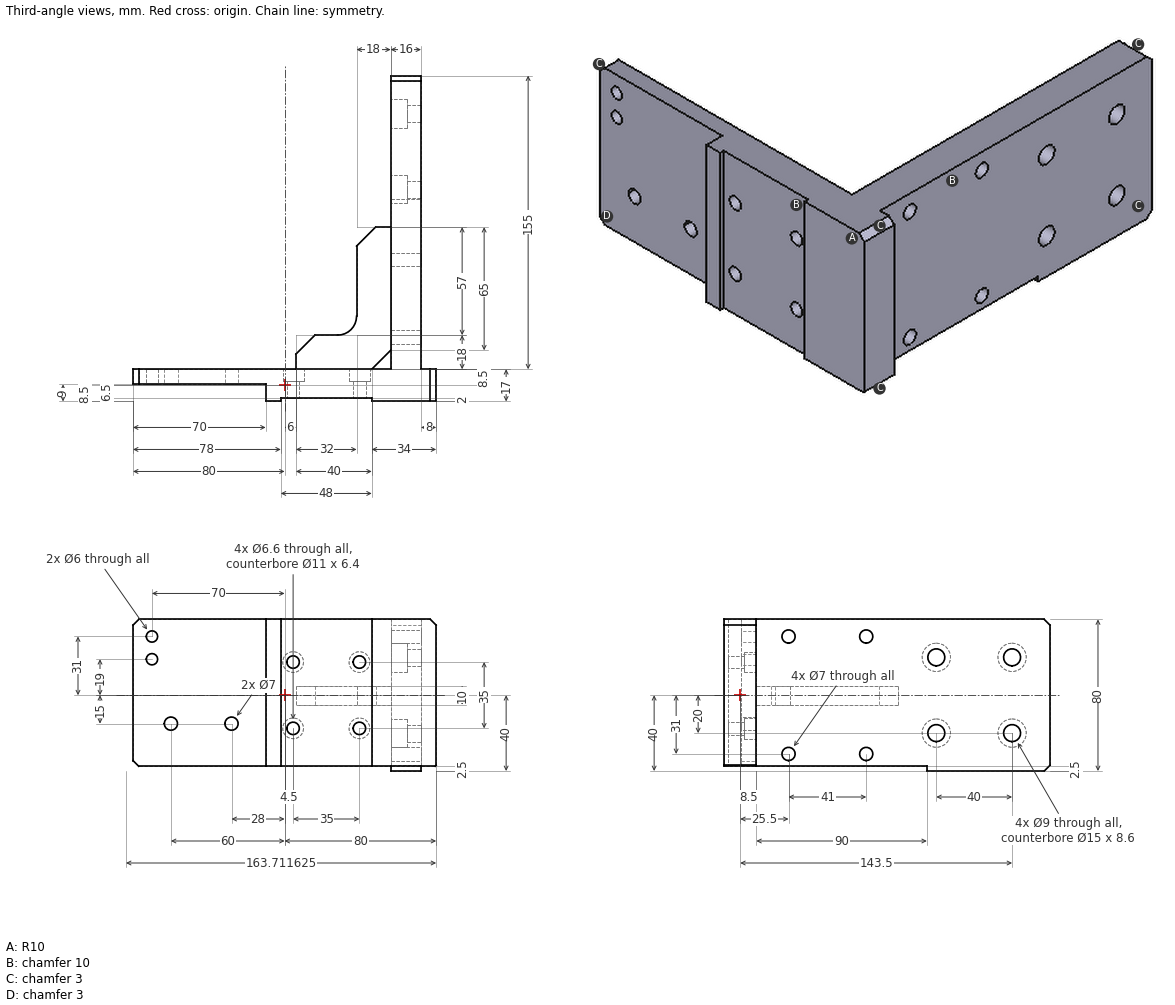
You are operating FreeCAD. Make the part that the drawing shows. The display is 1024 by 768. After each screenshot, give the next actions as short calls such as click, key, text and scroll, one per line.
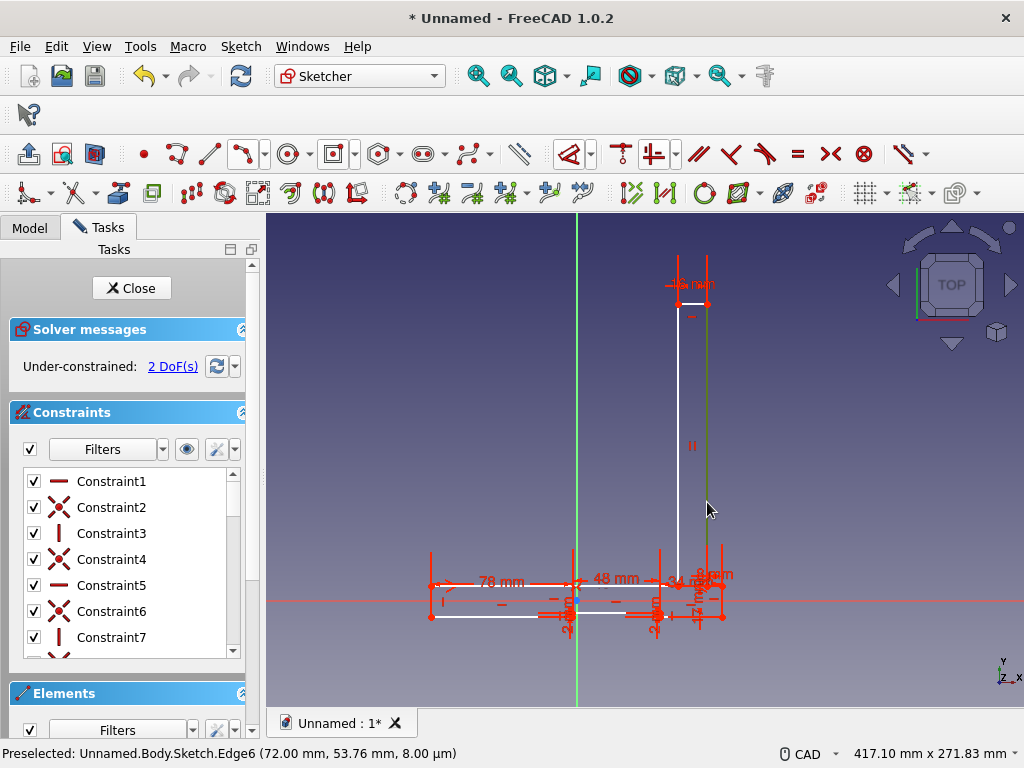
click(590, 154)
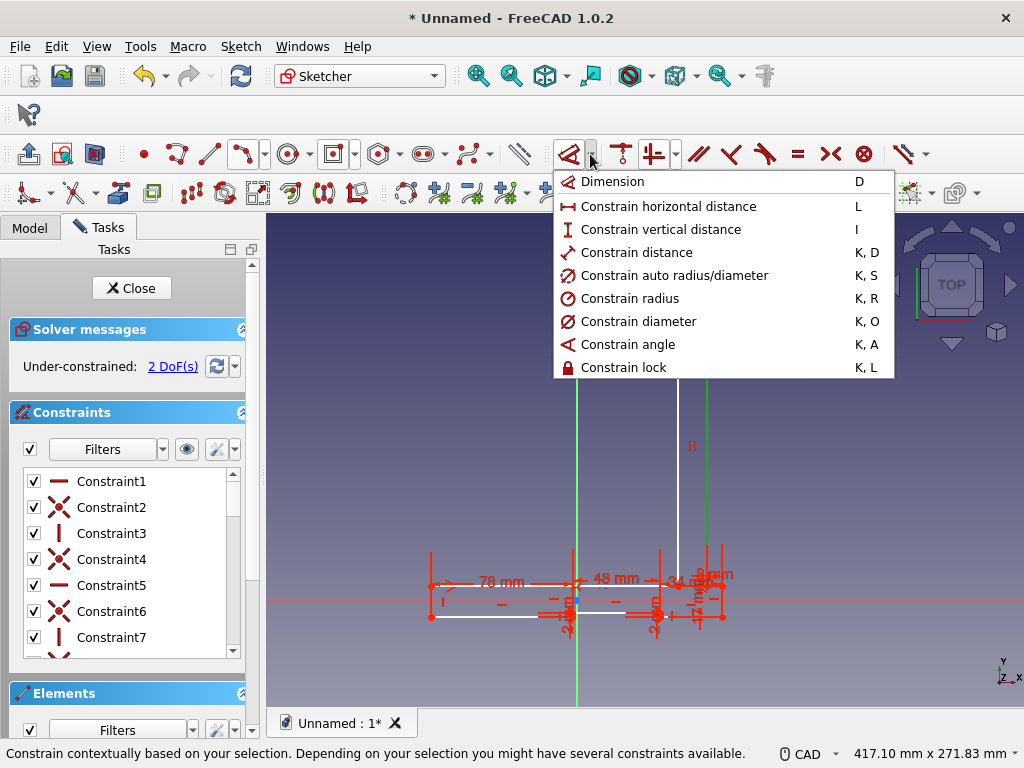
click(724, 230)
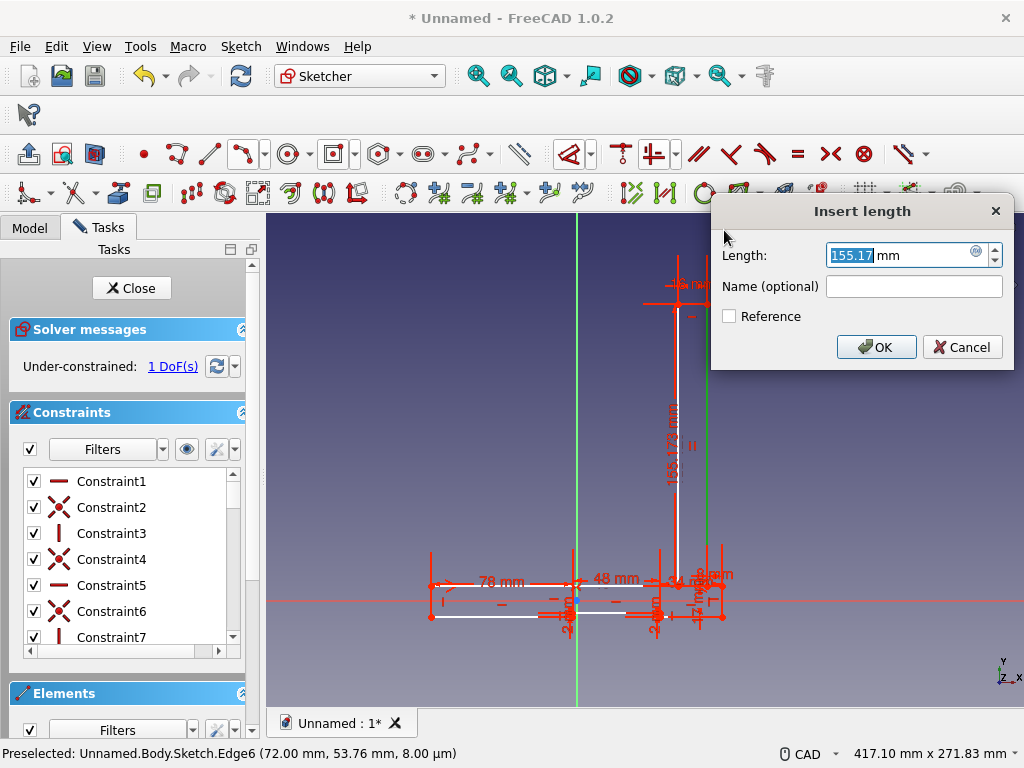
text(155)
key(Return)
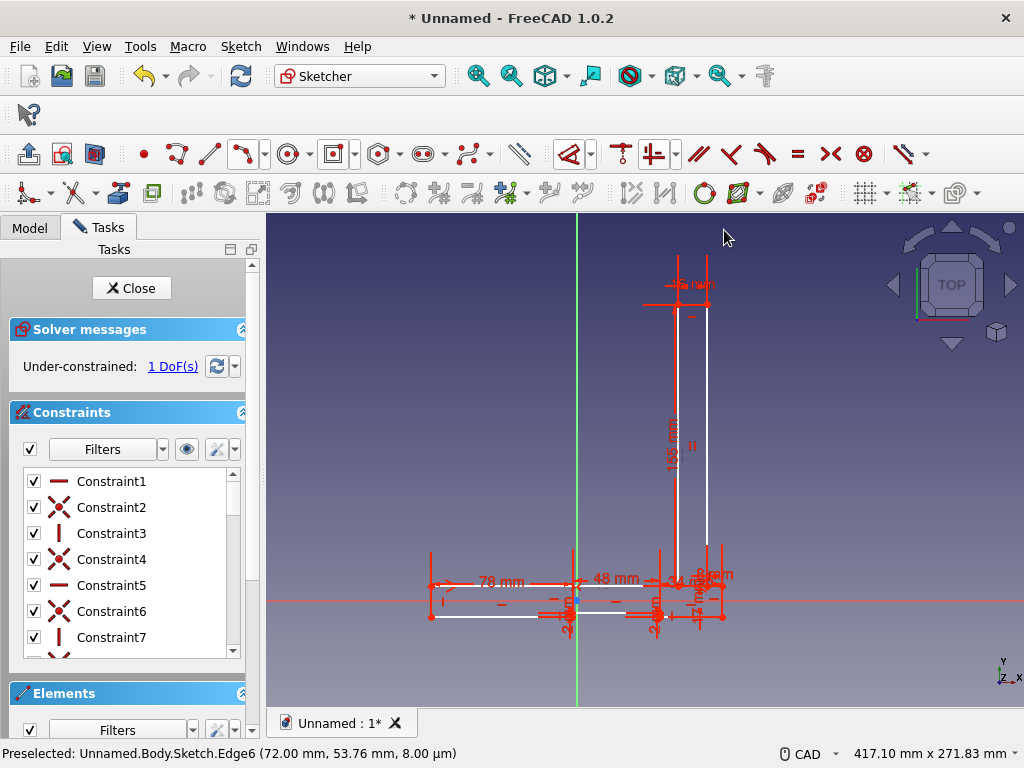
scroll(573, 613, up, 7)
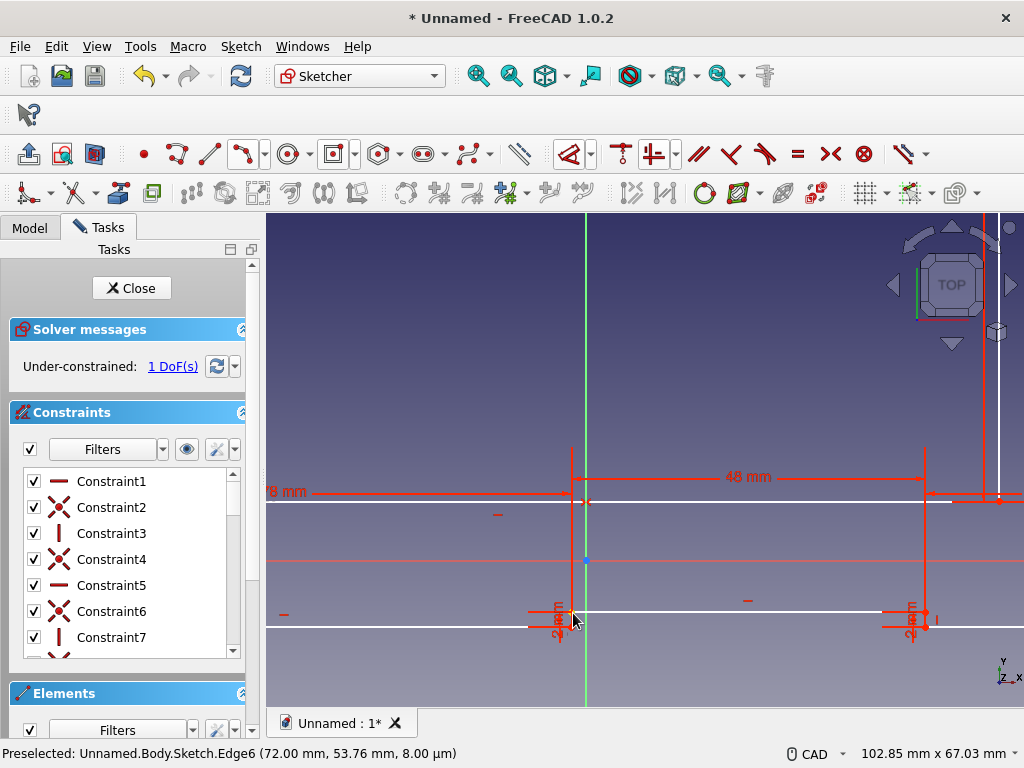
click(572, 612)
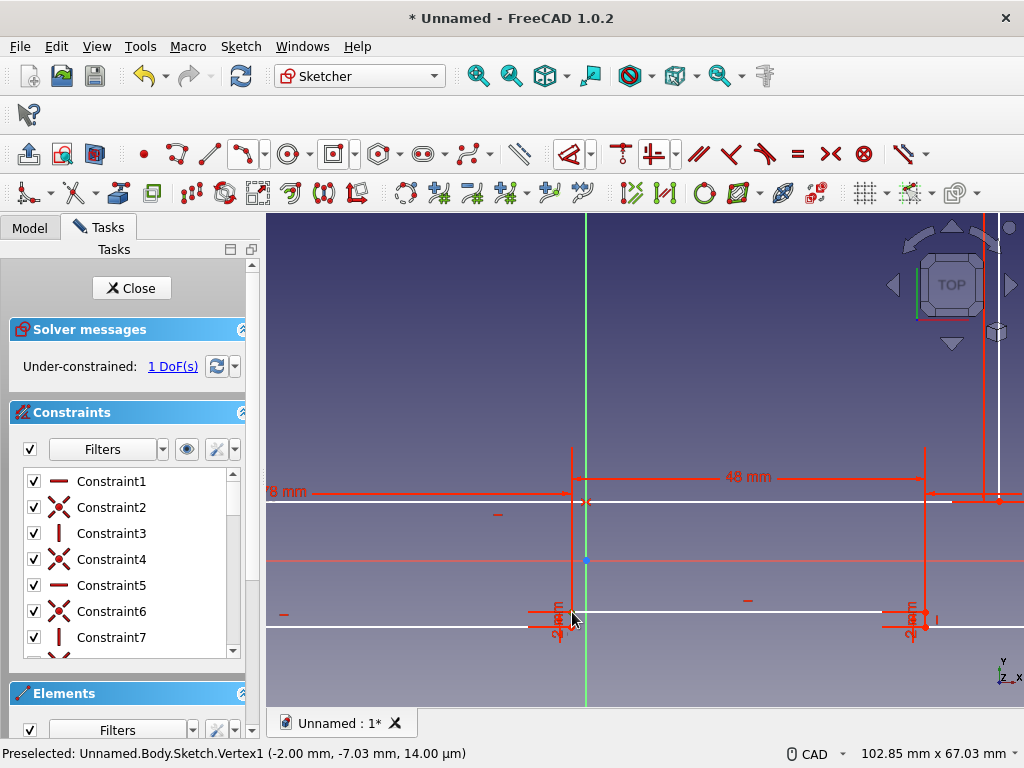
key(i)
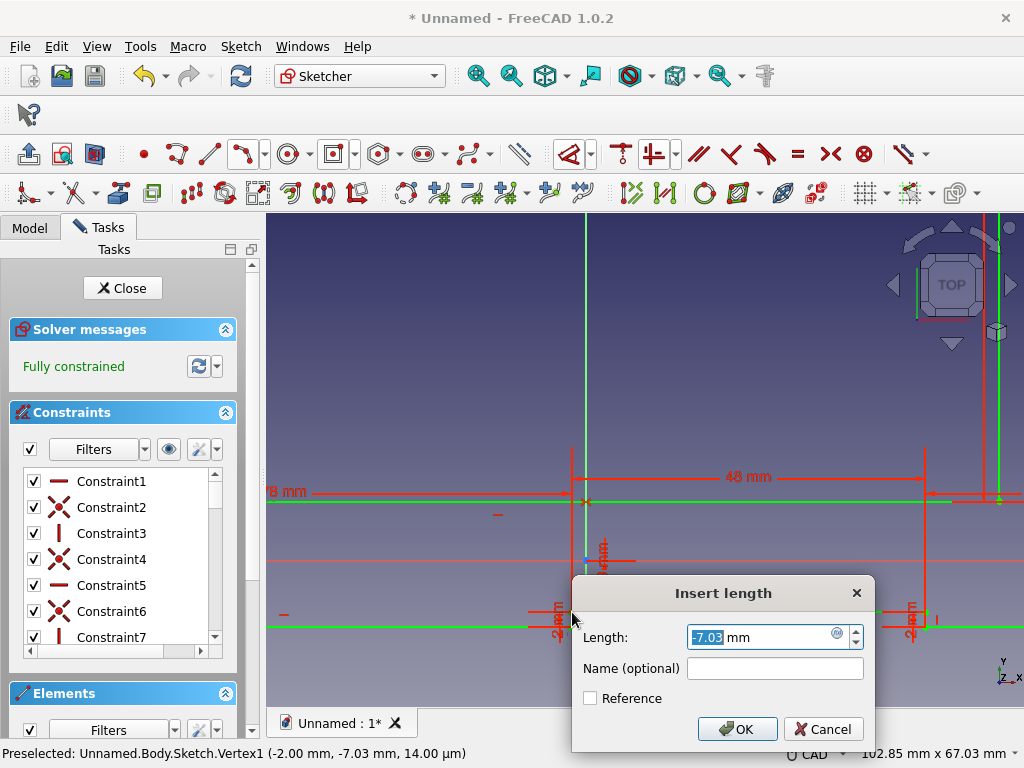
text(-6.5)
key(Return)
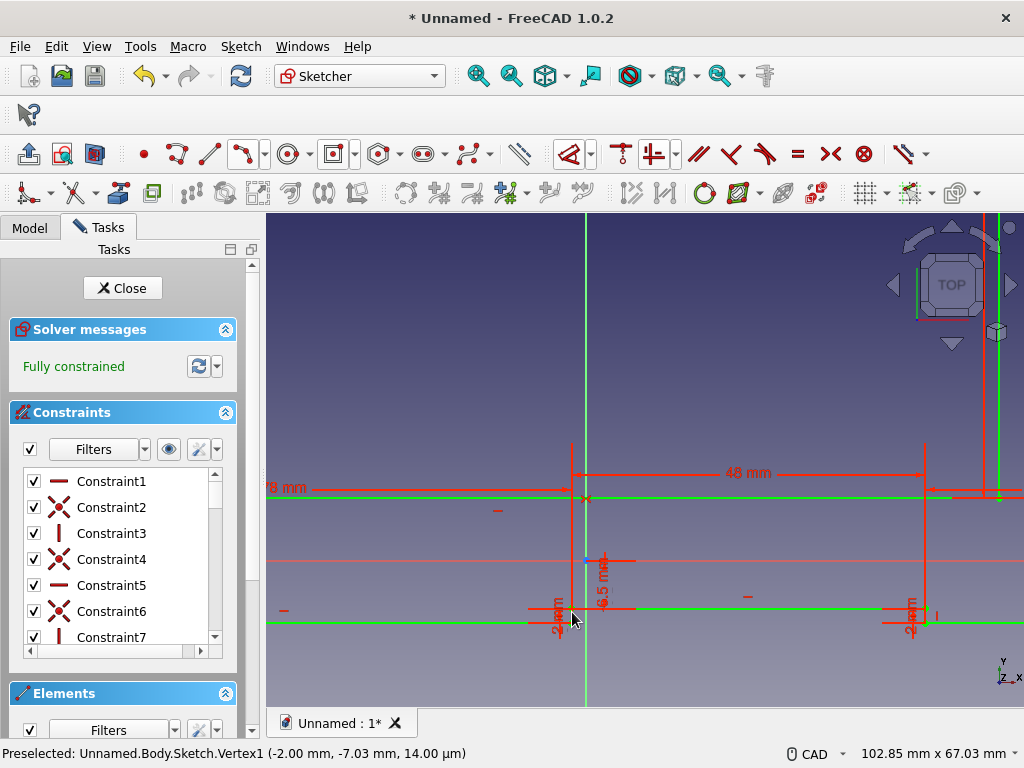
click(123, 288)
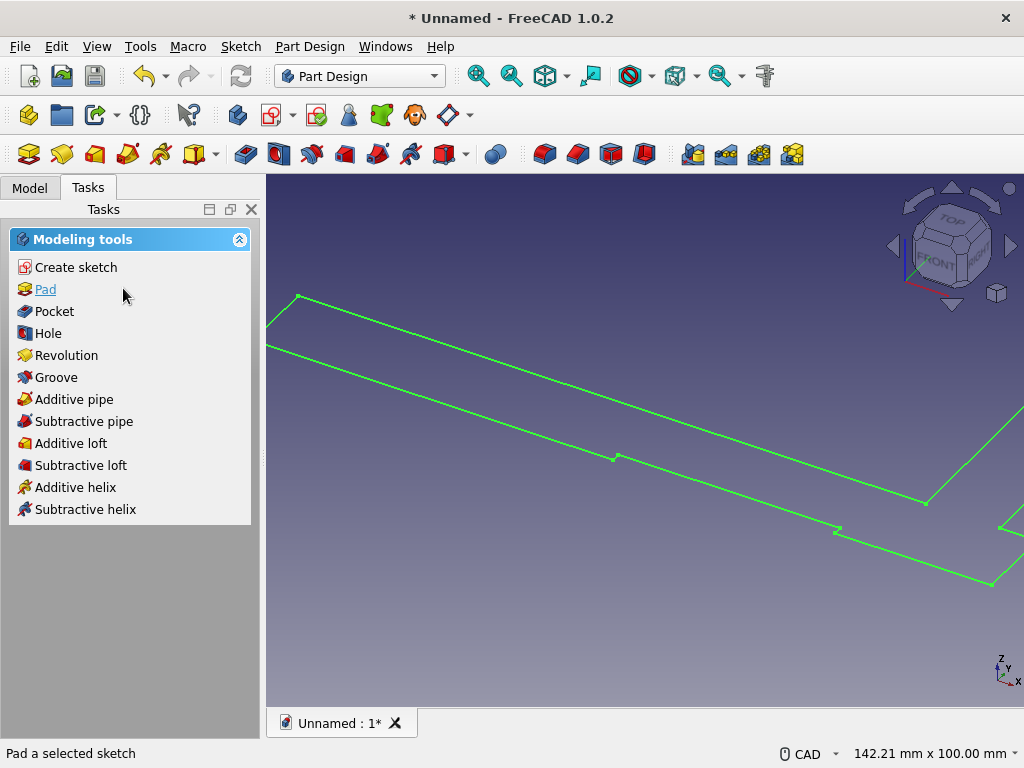
click(29, 154)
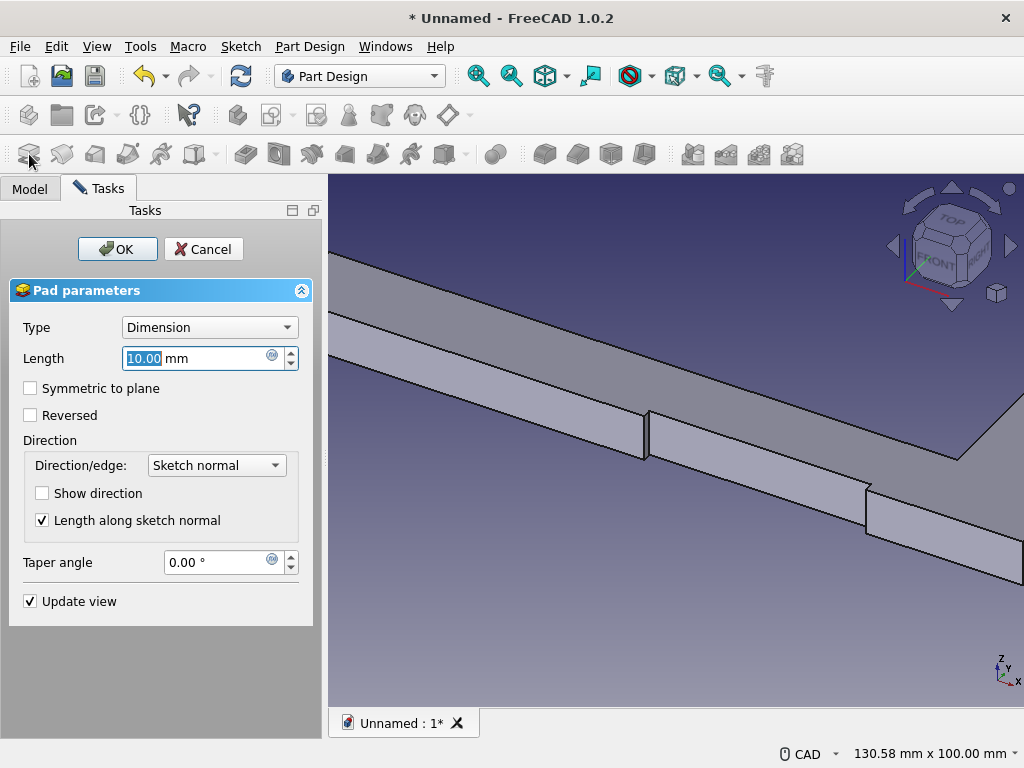
text(80)
key(Tab)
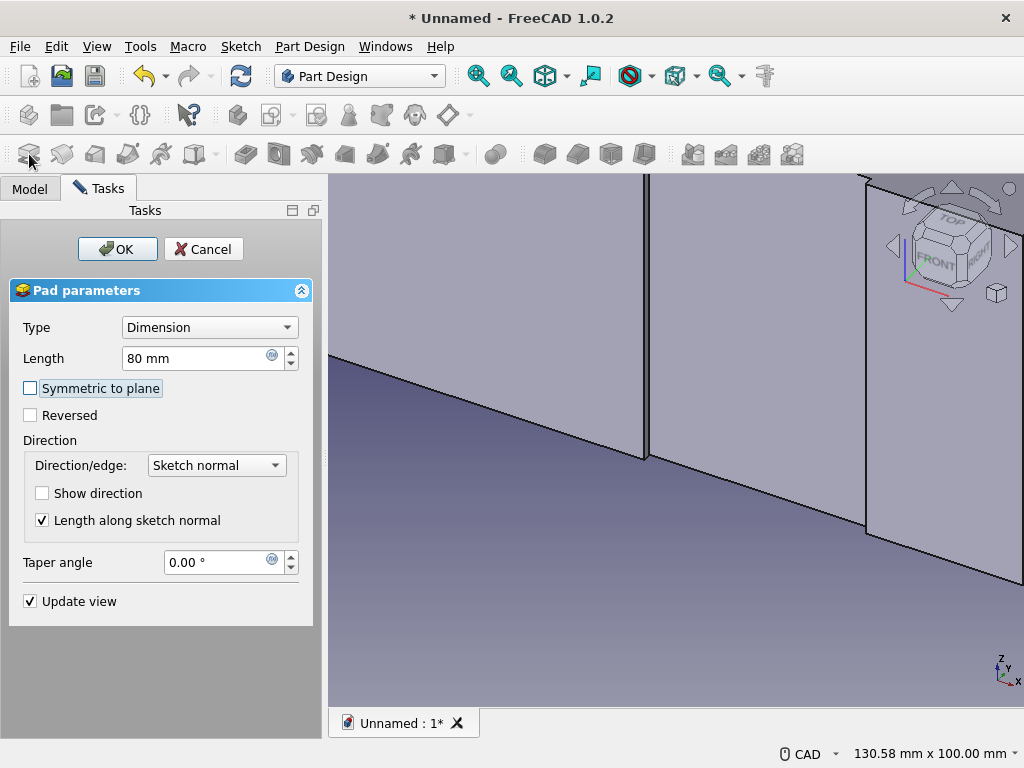
click(31, 388)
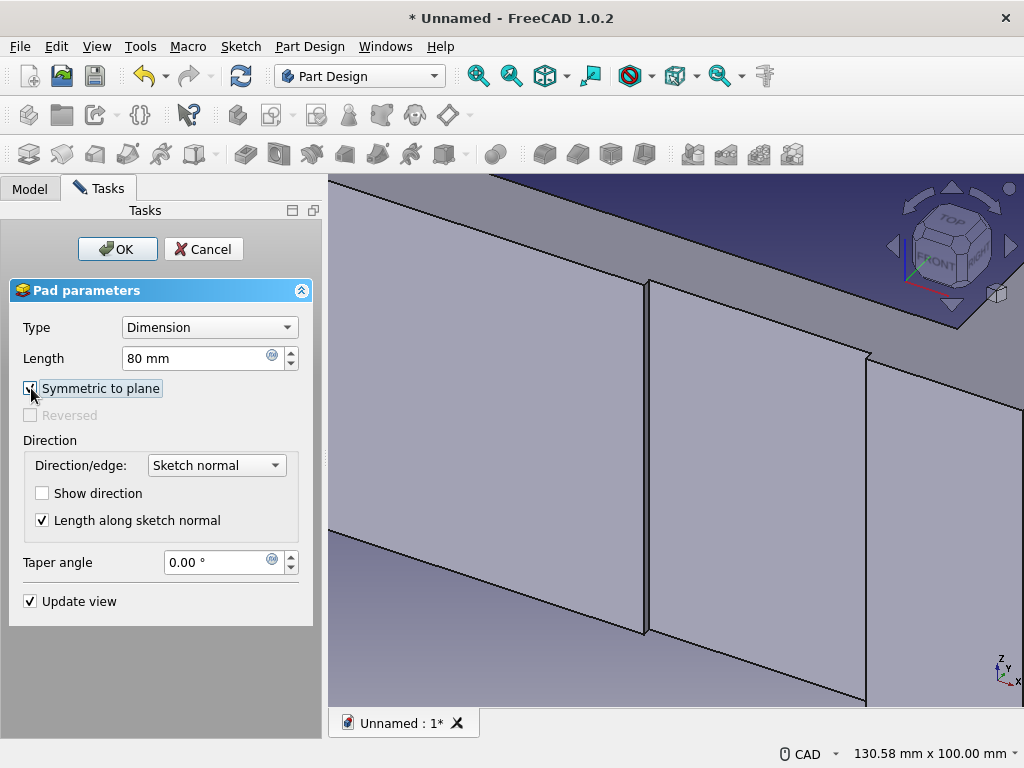
click(118, 249)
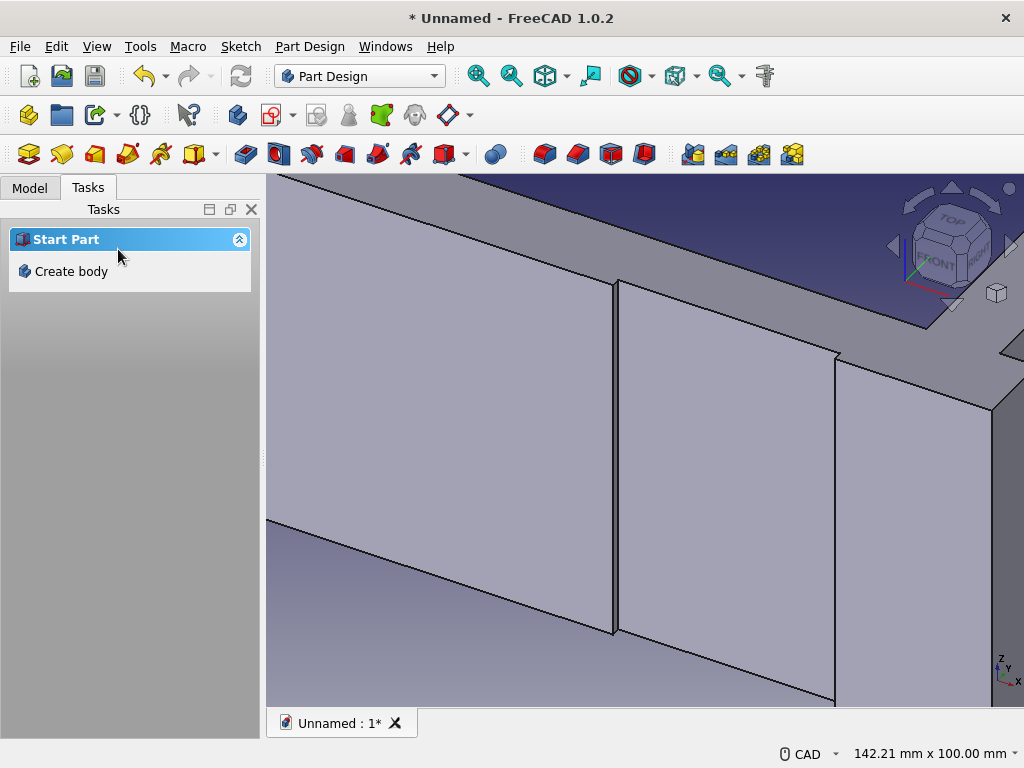
click(479, 76)